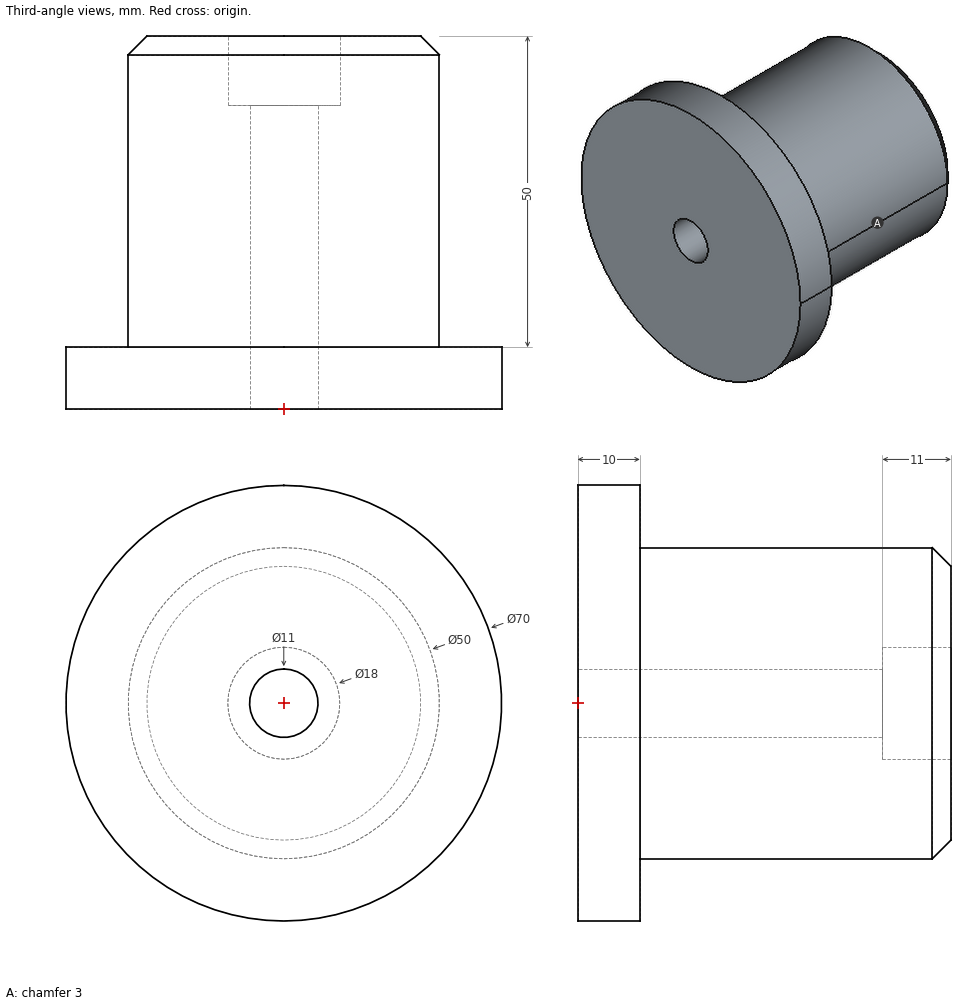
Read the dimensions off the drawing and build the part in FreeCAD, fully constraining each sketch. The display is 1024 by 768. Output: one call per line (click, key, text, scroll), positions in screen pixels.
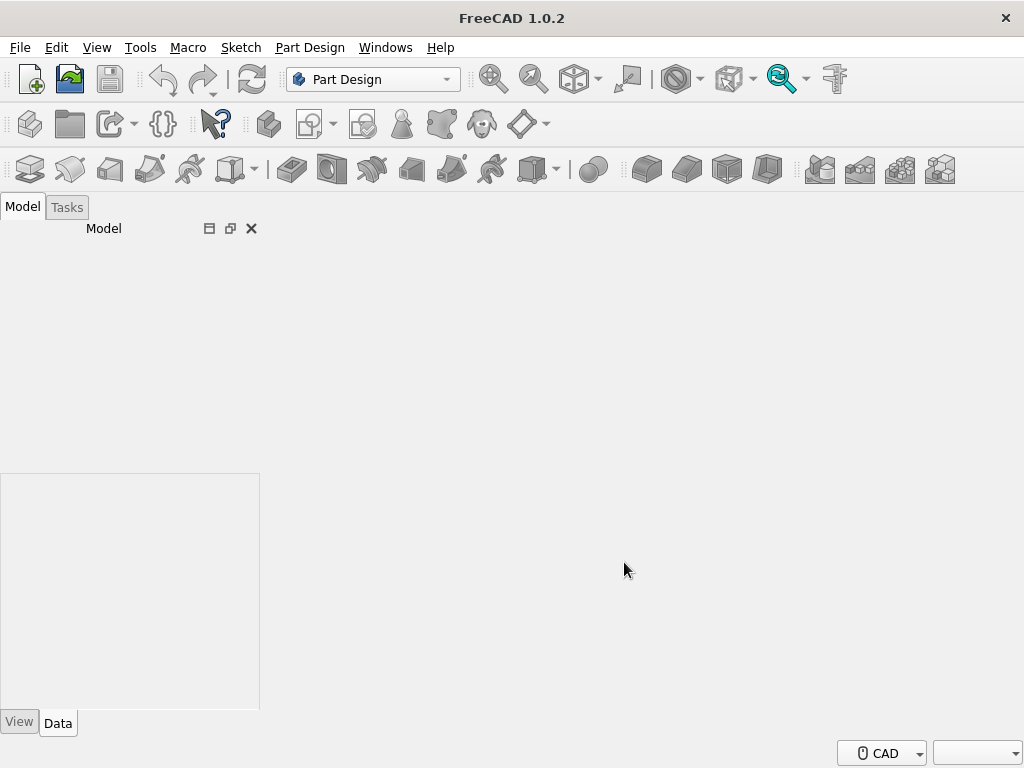
key(ctrl+n)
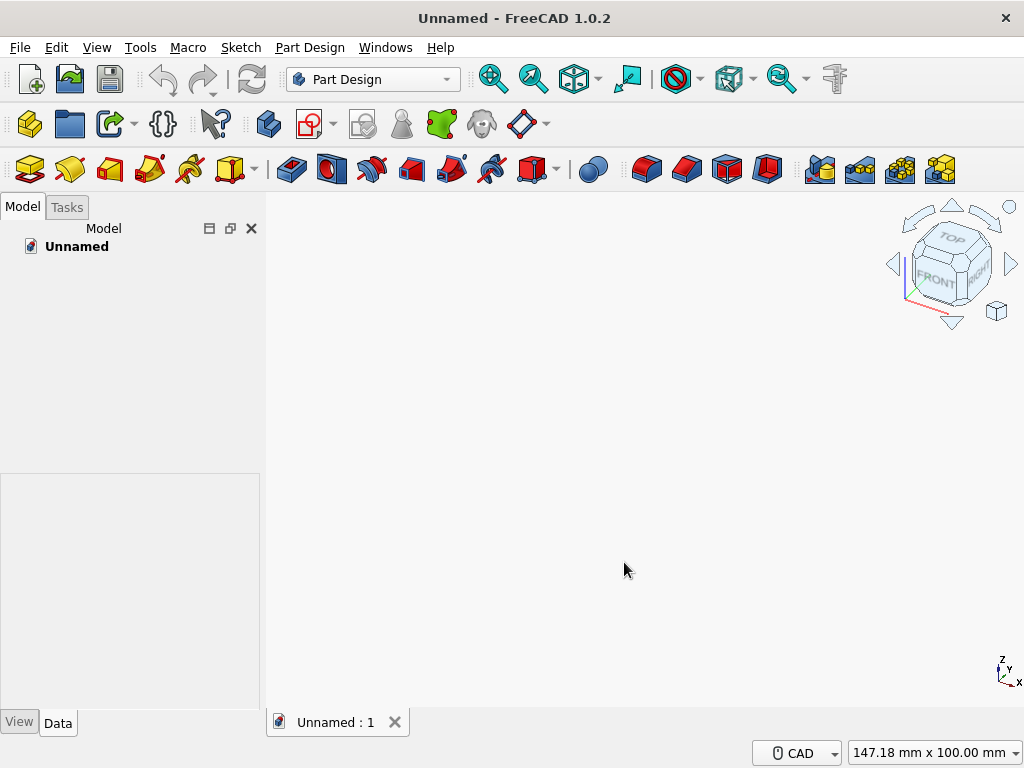
click(310, 124)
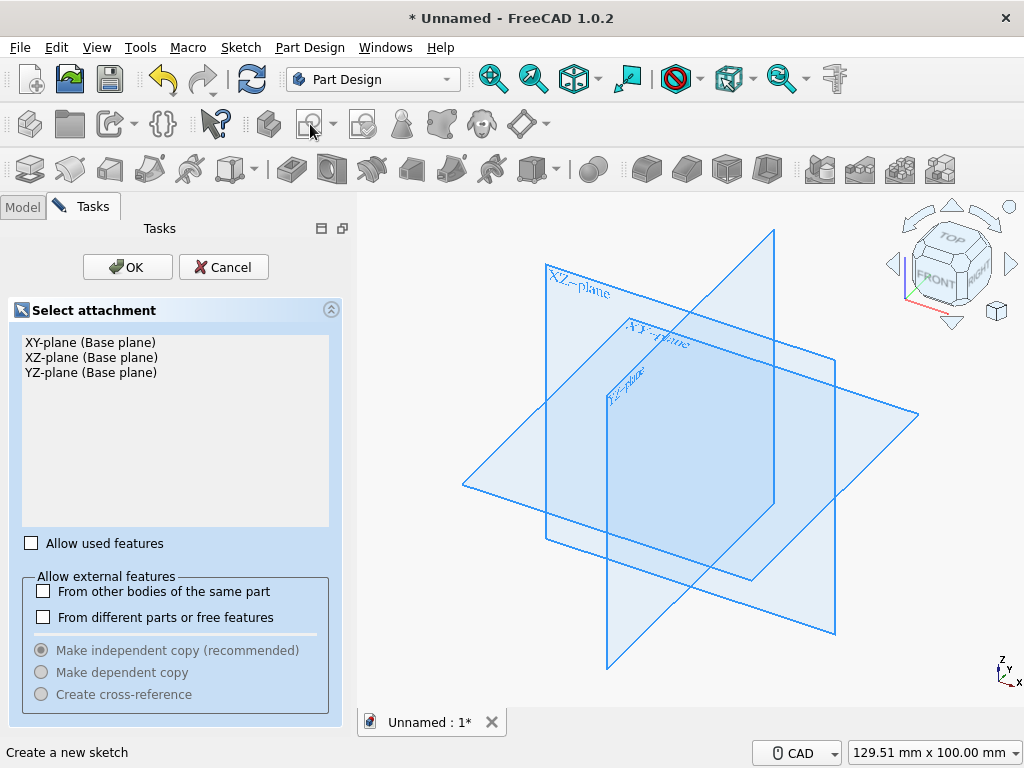
click(82, 358)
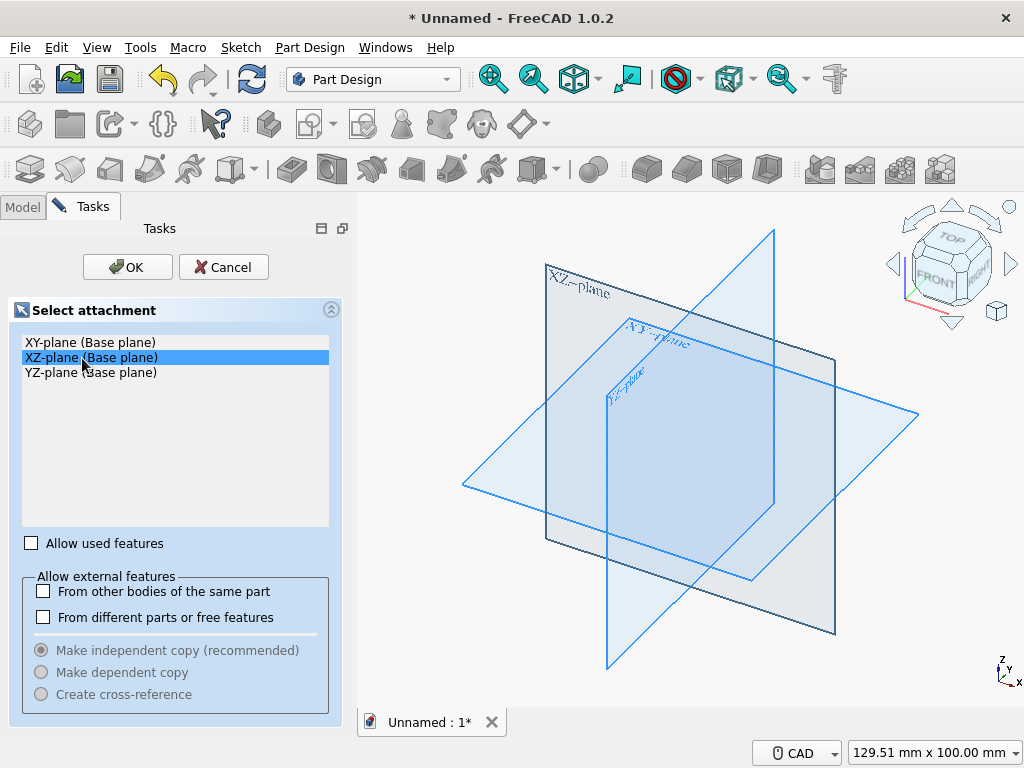
click(128, 267)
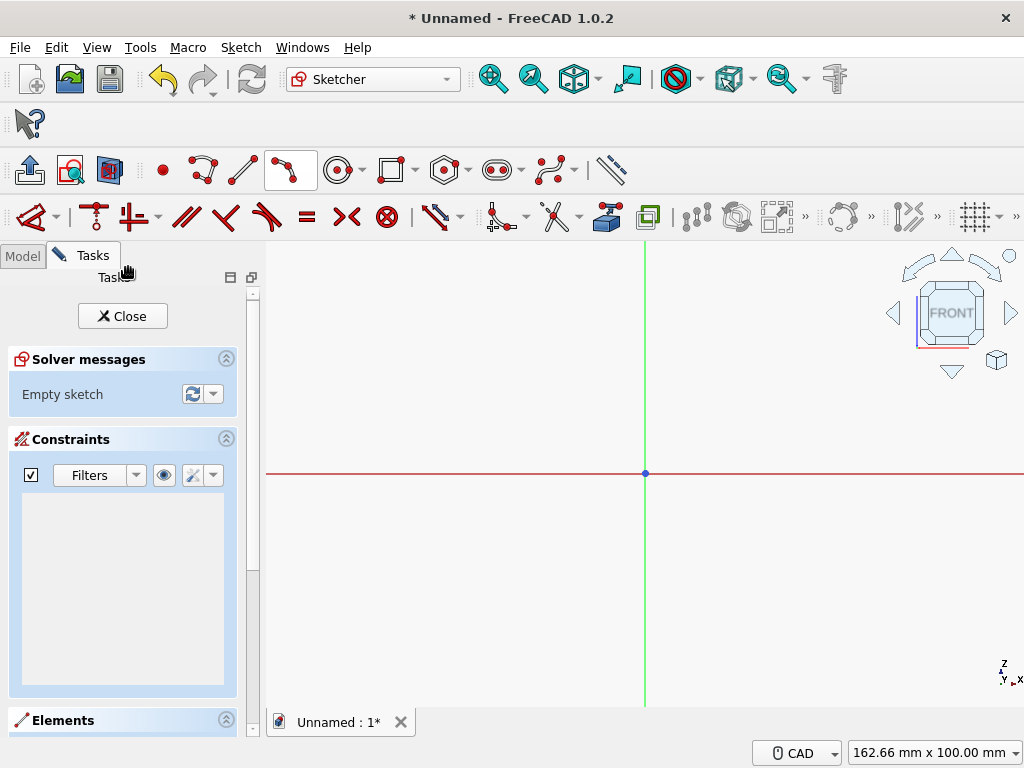
key(g)
key(c)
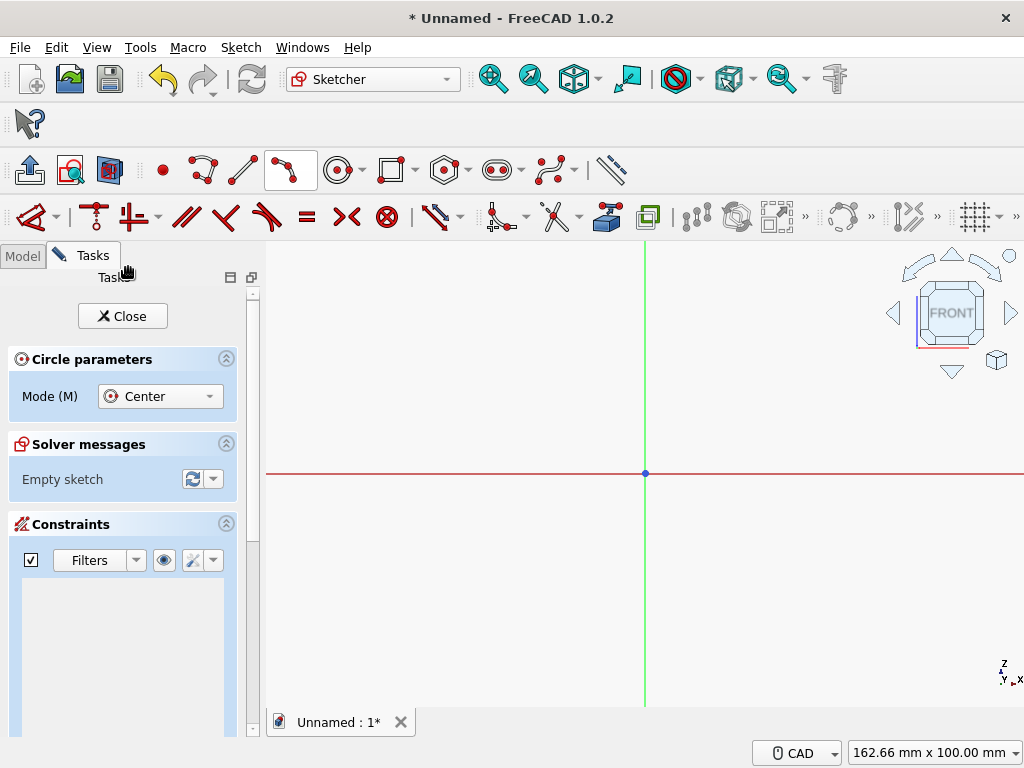
click(645, 474)
move(760, 359)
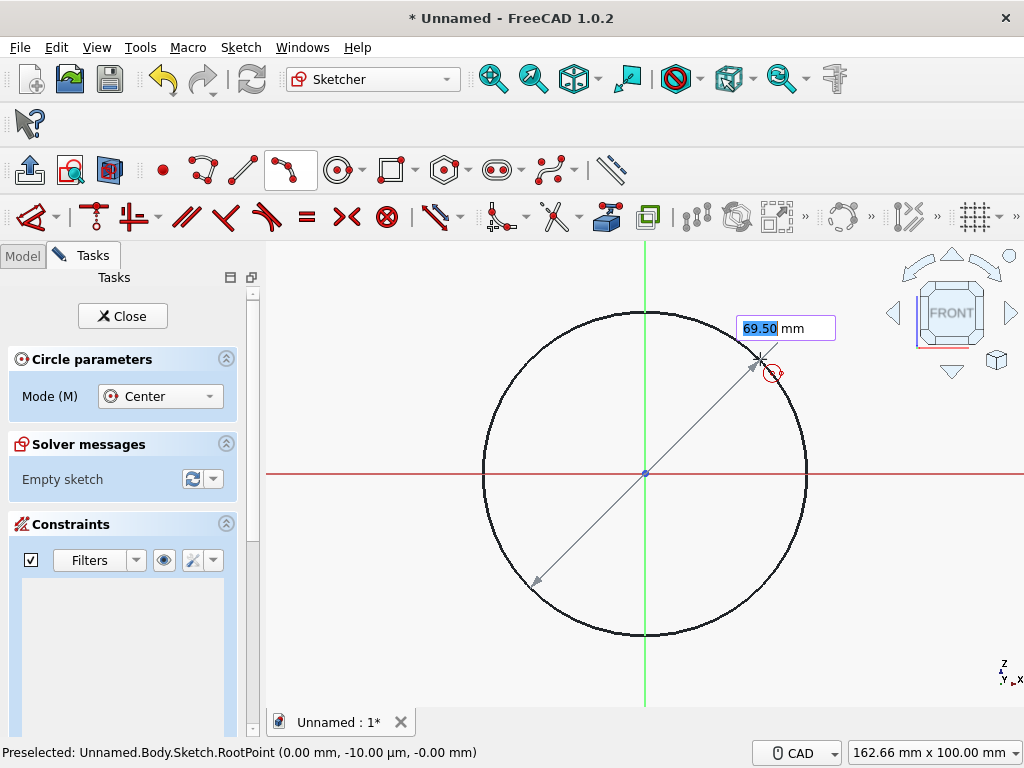
text(70)
key(Return)
key(Escape)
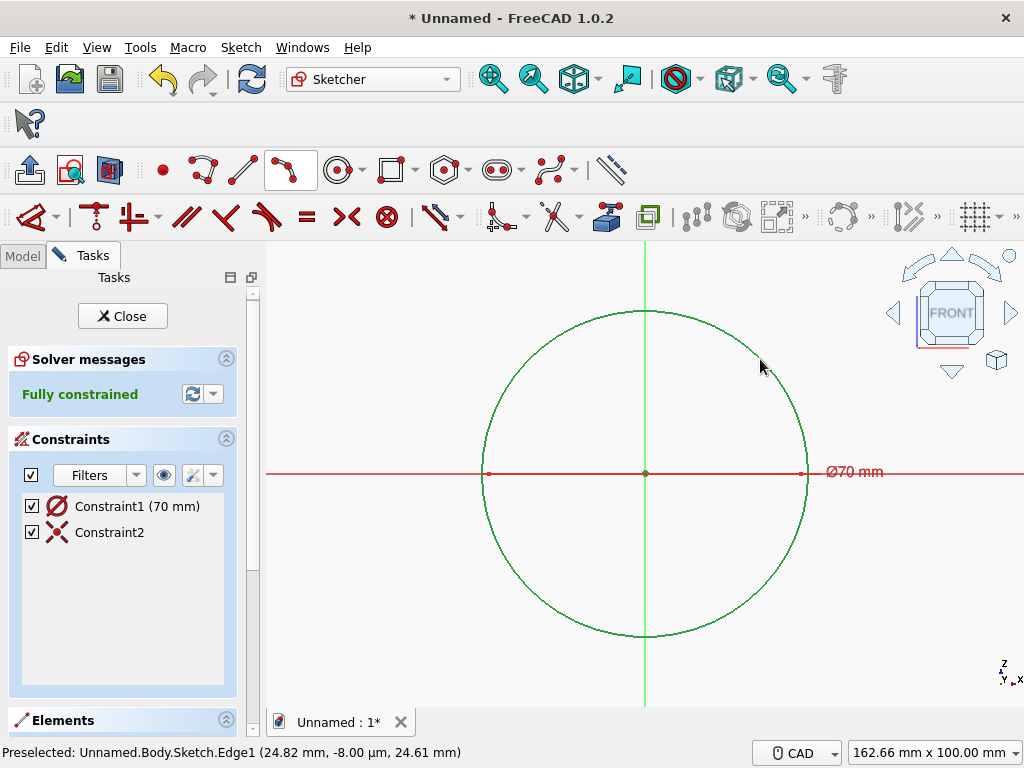
click(123, 316)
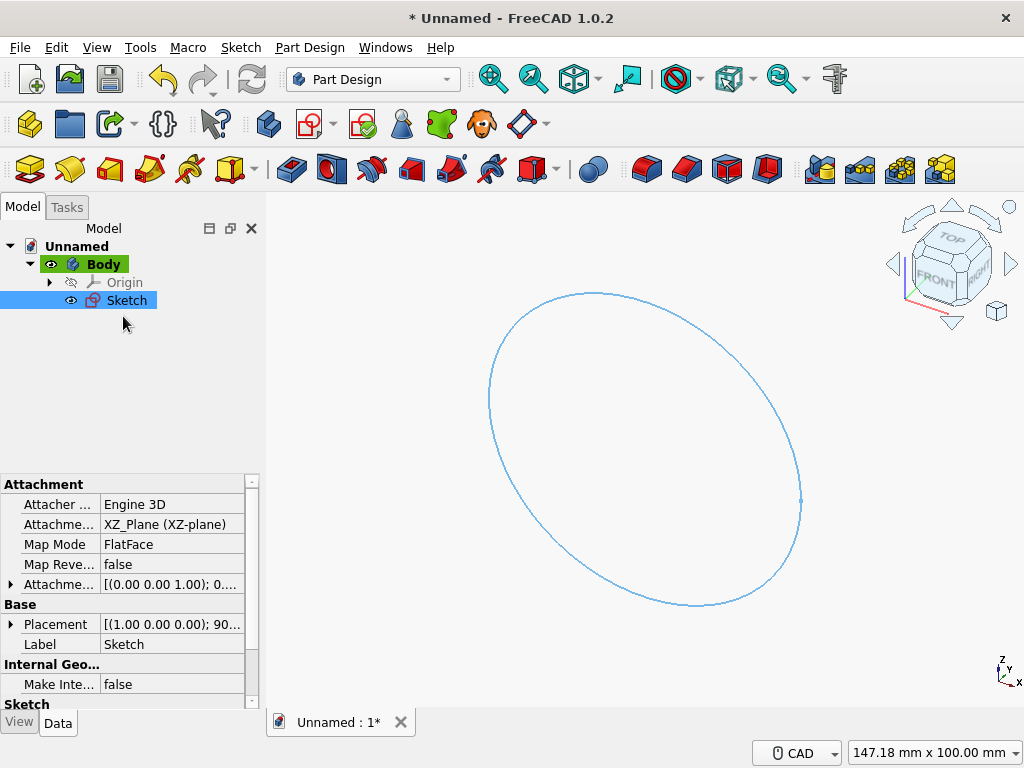
click(30, 170)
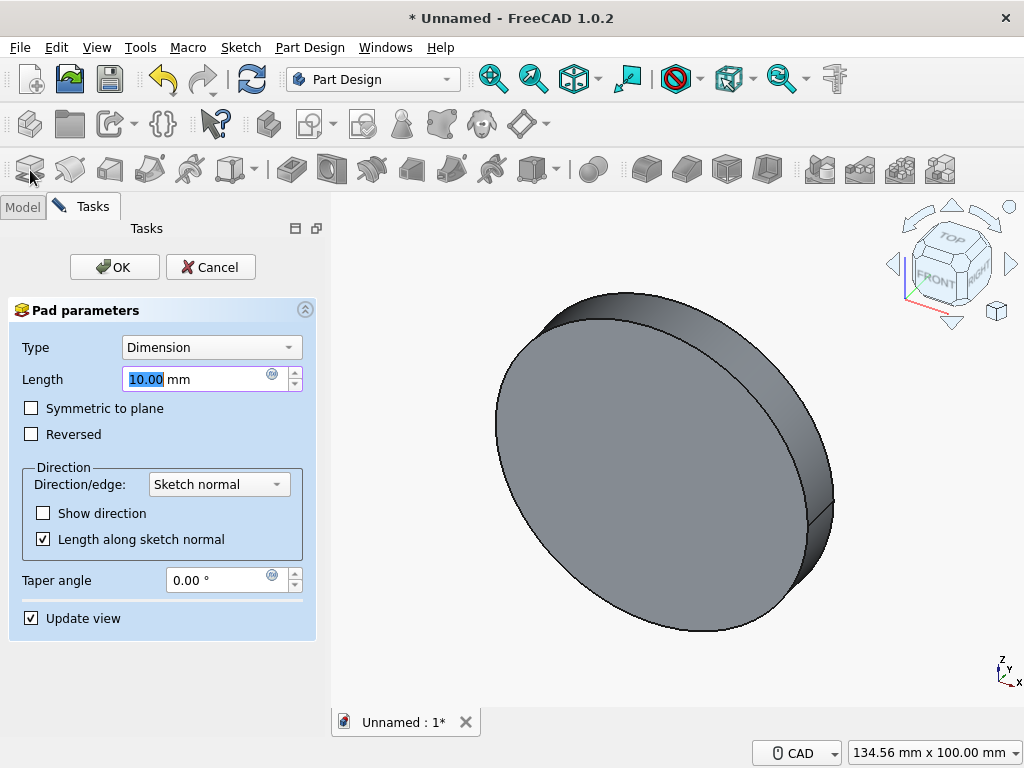
text(10)
key(Tab)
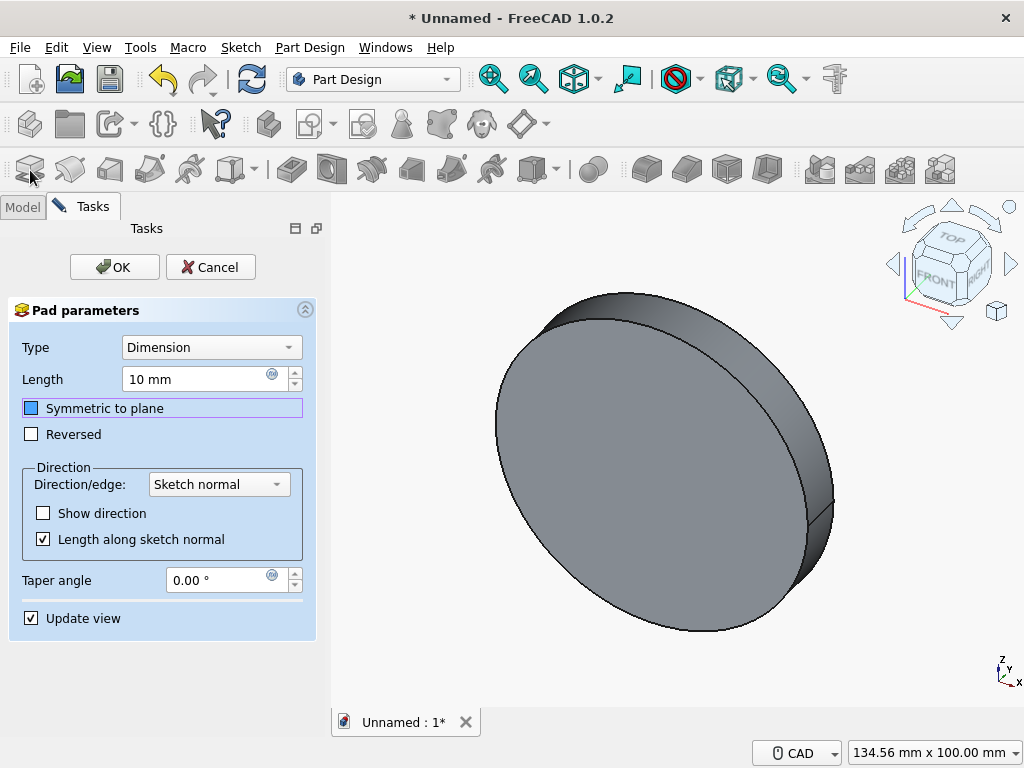
click(30, 434)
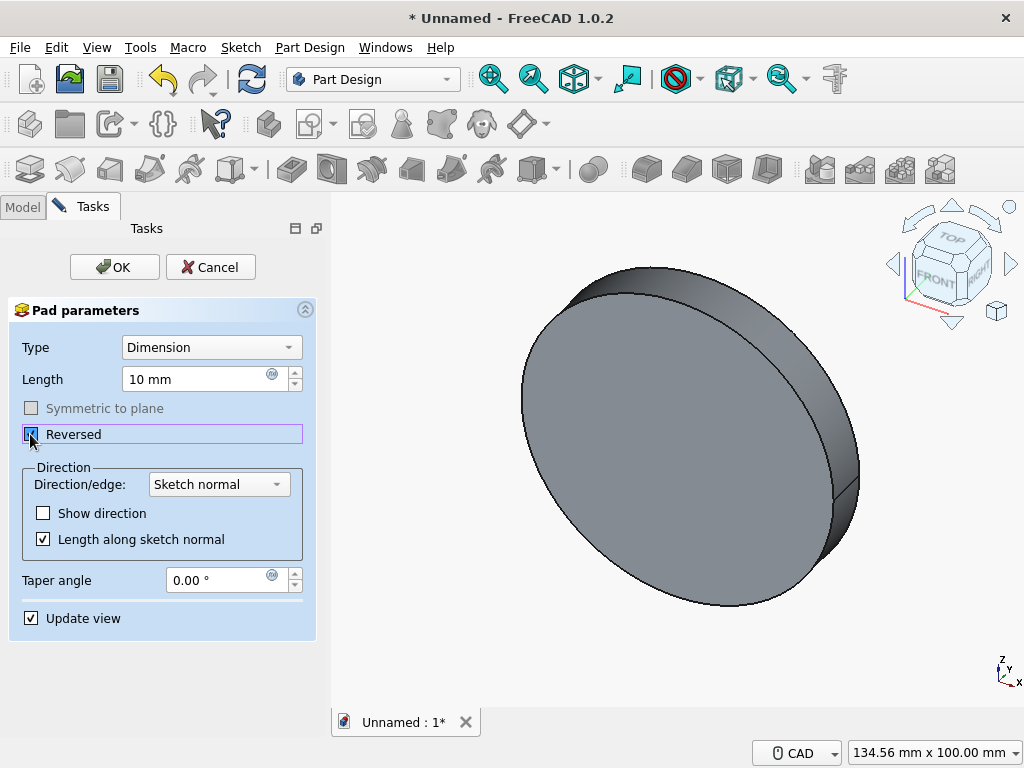
click(115, 267)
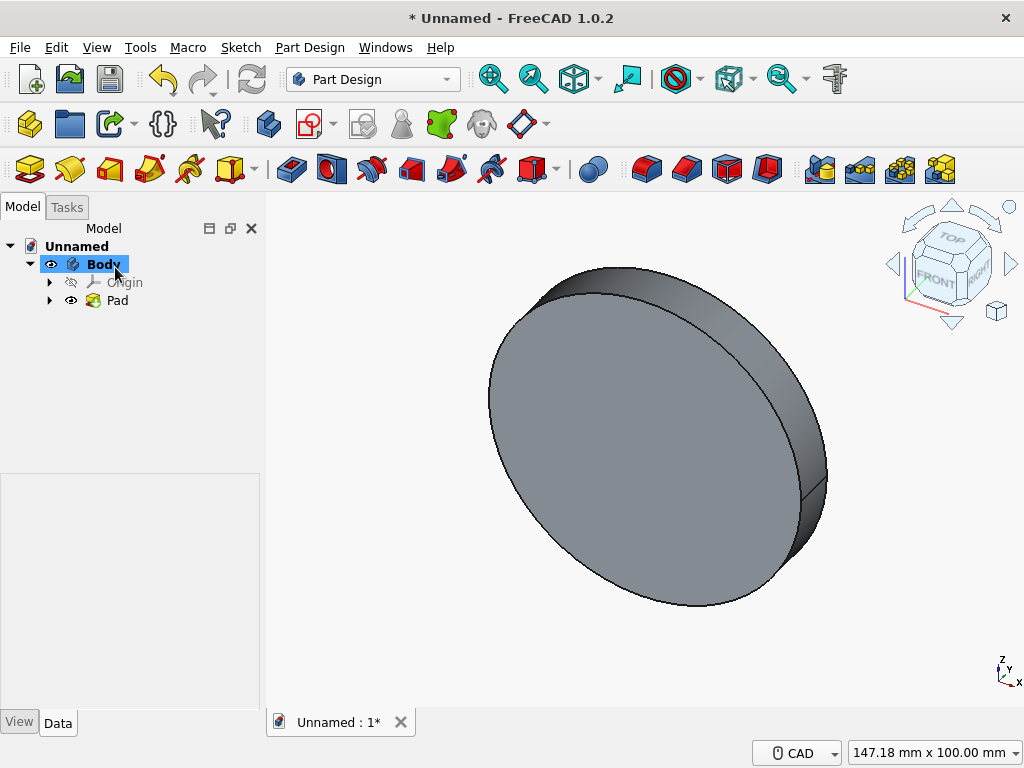
key(4)